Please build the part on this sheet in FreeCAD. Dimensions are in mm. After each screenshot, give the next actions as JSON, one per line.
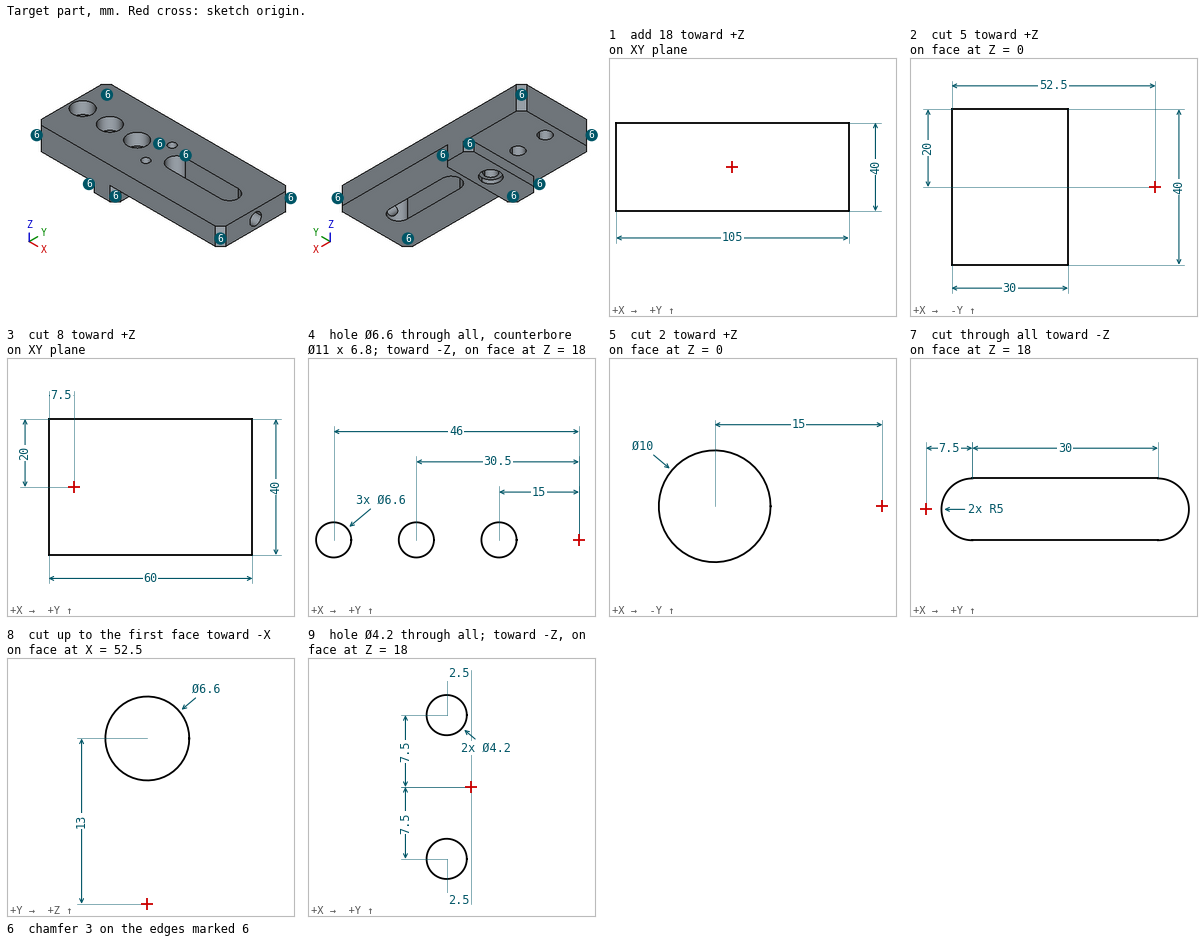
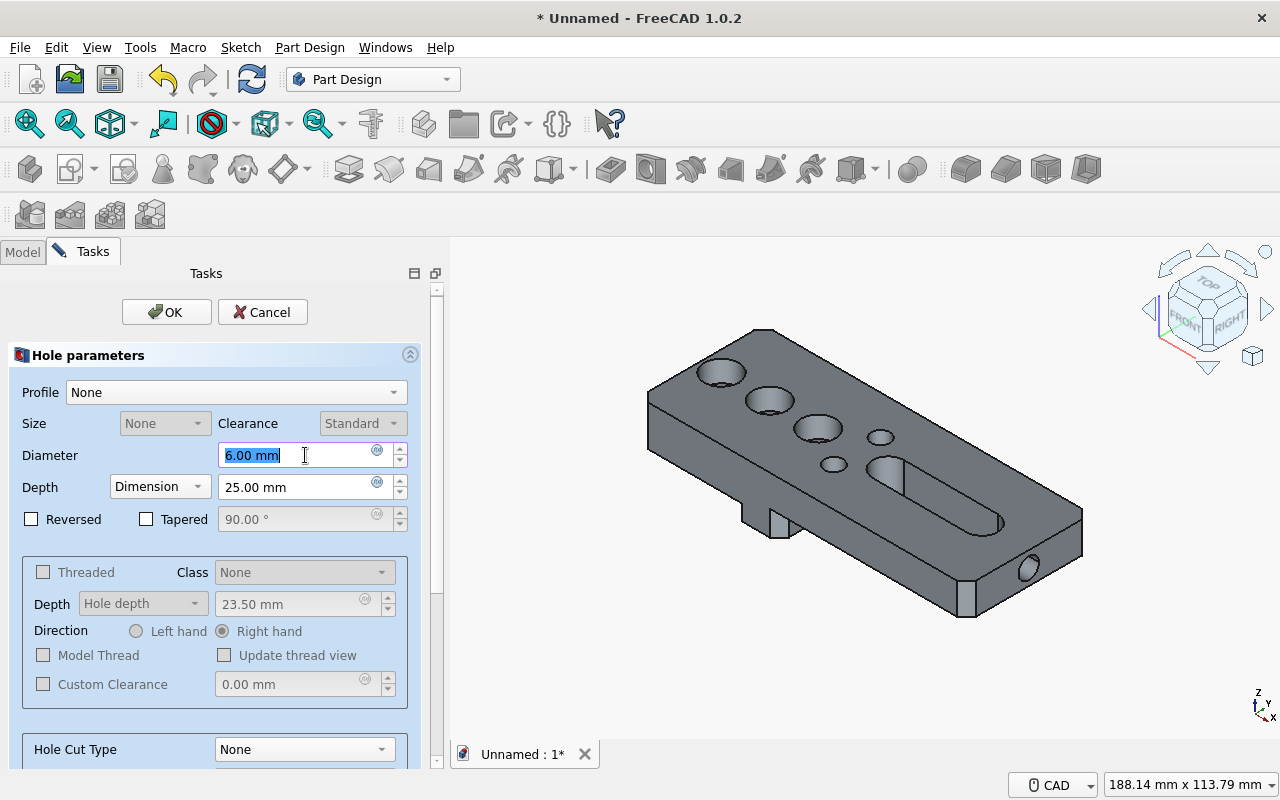
{"action": "type", "text": "4.2"}
{"action": "key", "text": "Tab"}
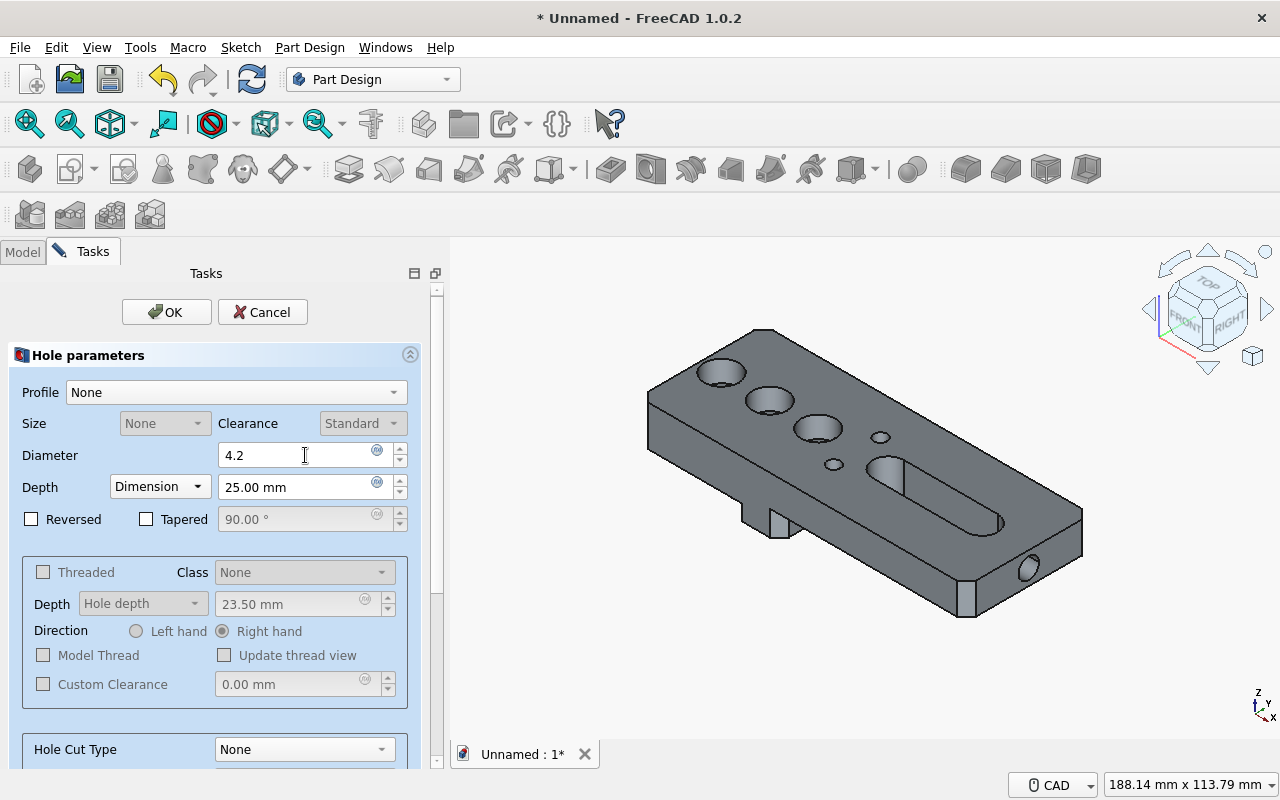
{"action": "left_click", "coordinate": [161, 486]}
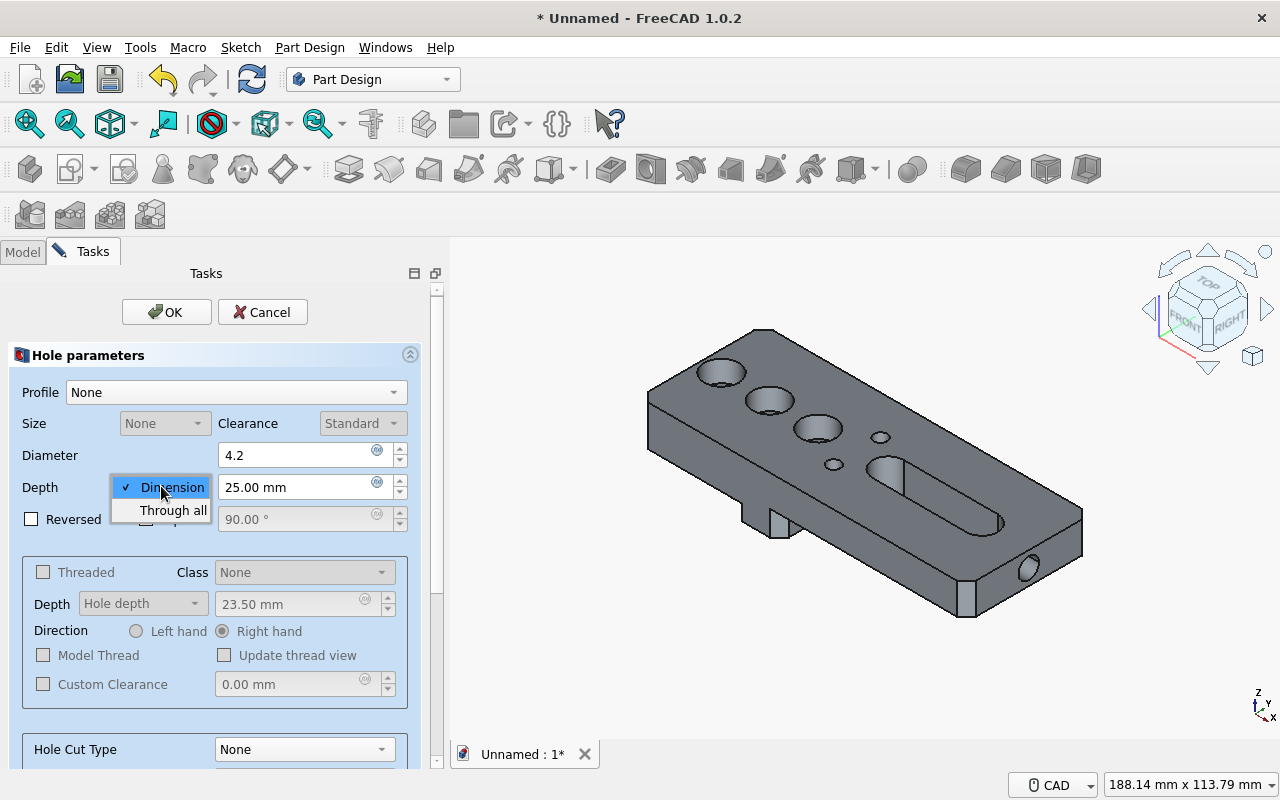
{"action": "left_click", "coordinate": [160, 510]}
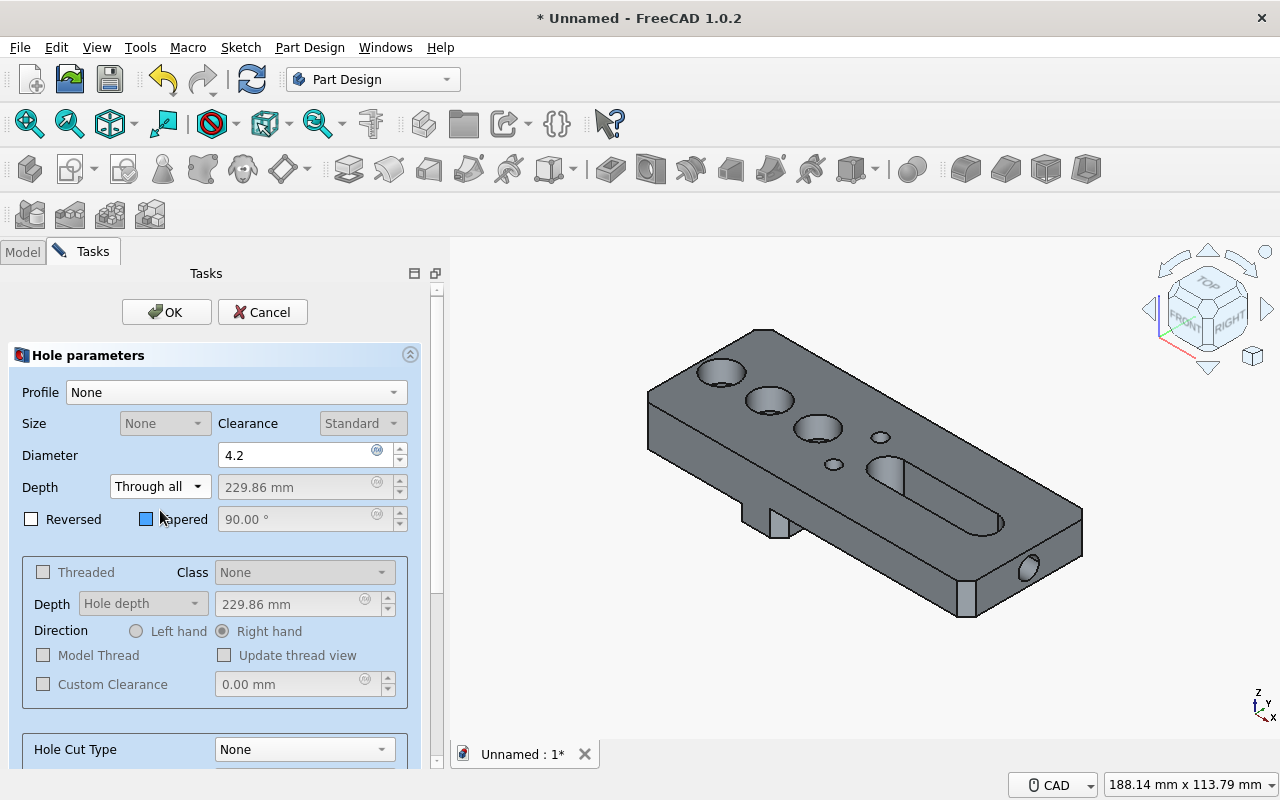
{"action": "left_click", "coordinate": [167, 312]}